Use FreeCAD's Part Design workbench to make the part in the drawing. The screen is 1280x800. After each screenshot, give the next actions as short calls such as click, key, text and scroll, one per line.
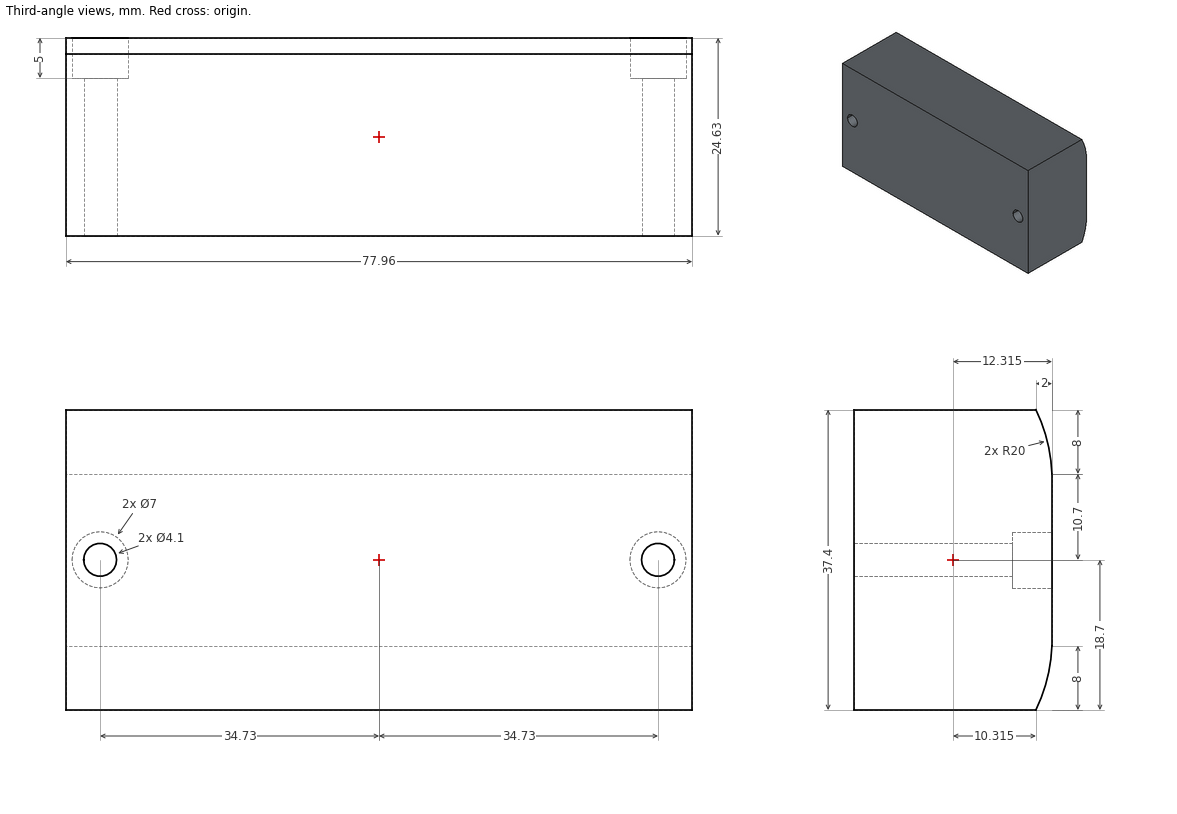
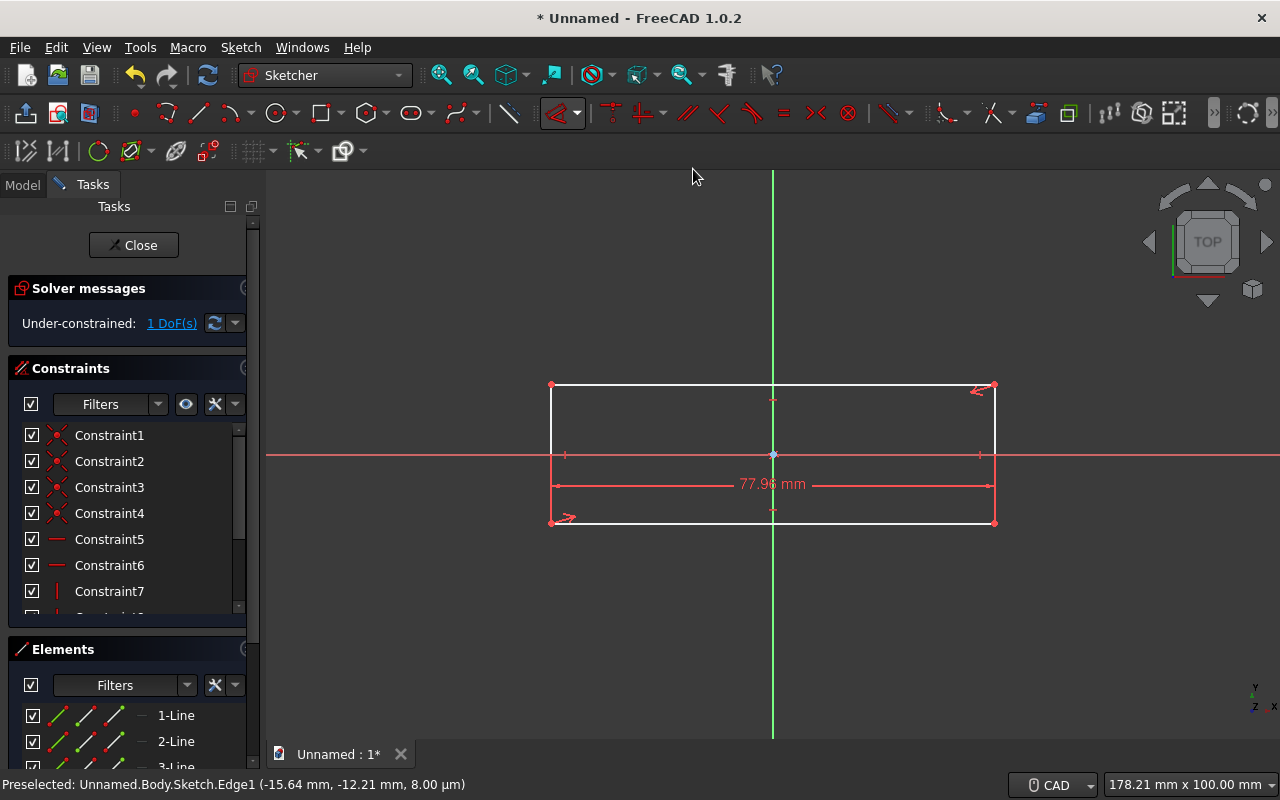
click(995, 482)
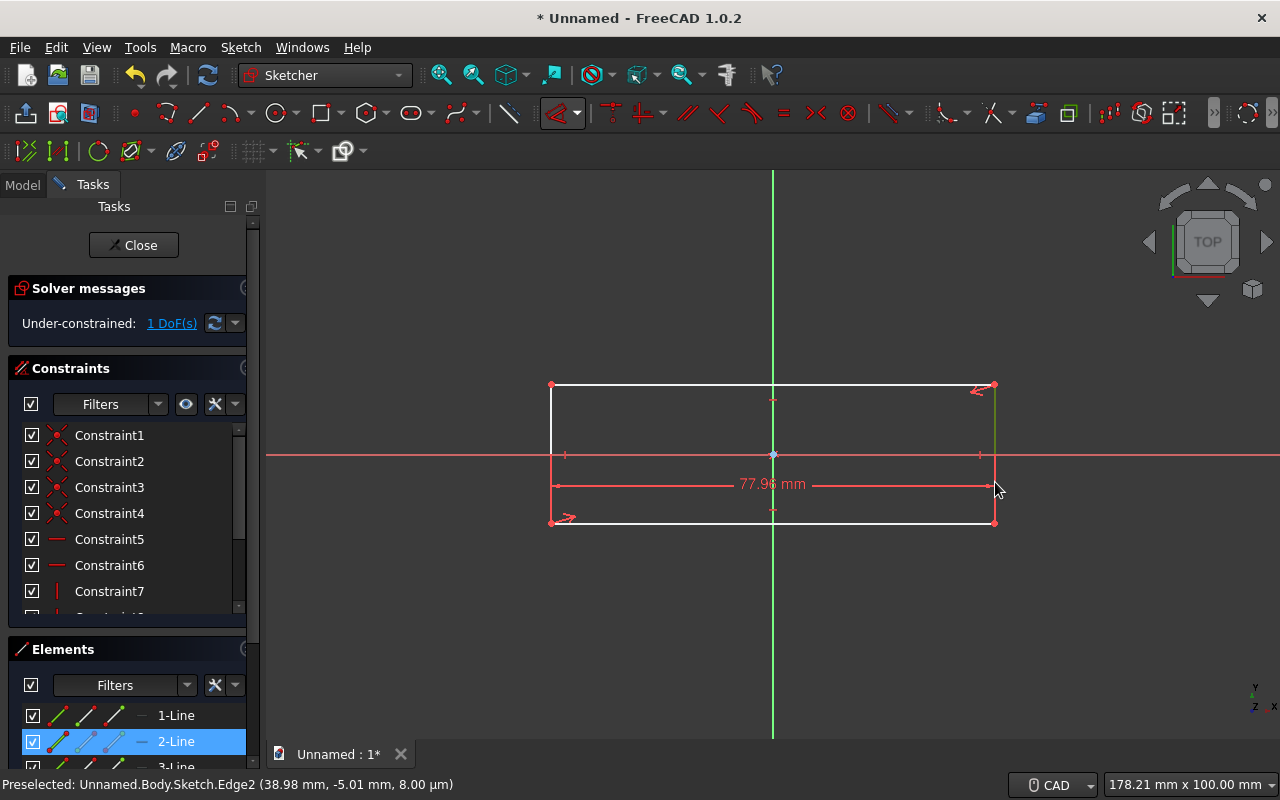
click(580, 114)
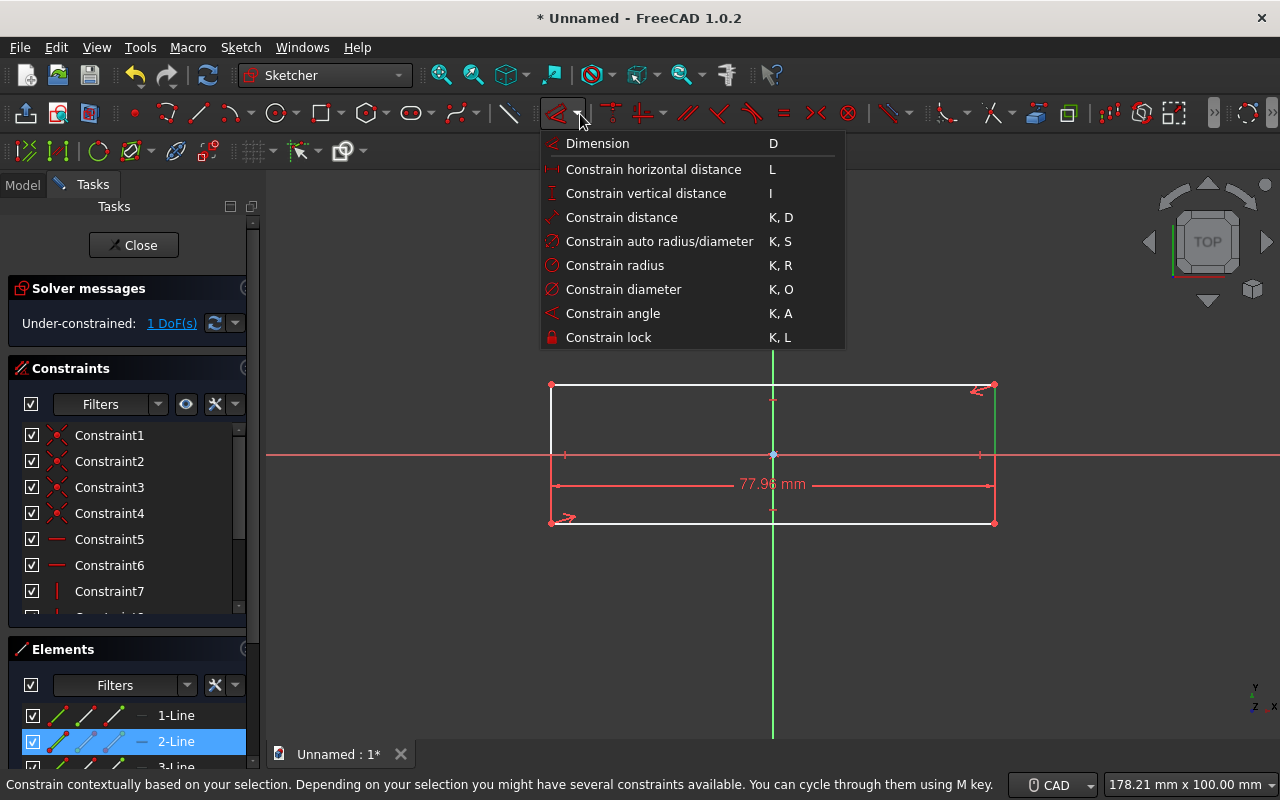
click(693, 193)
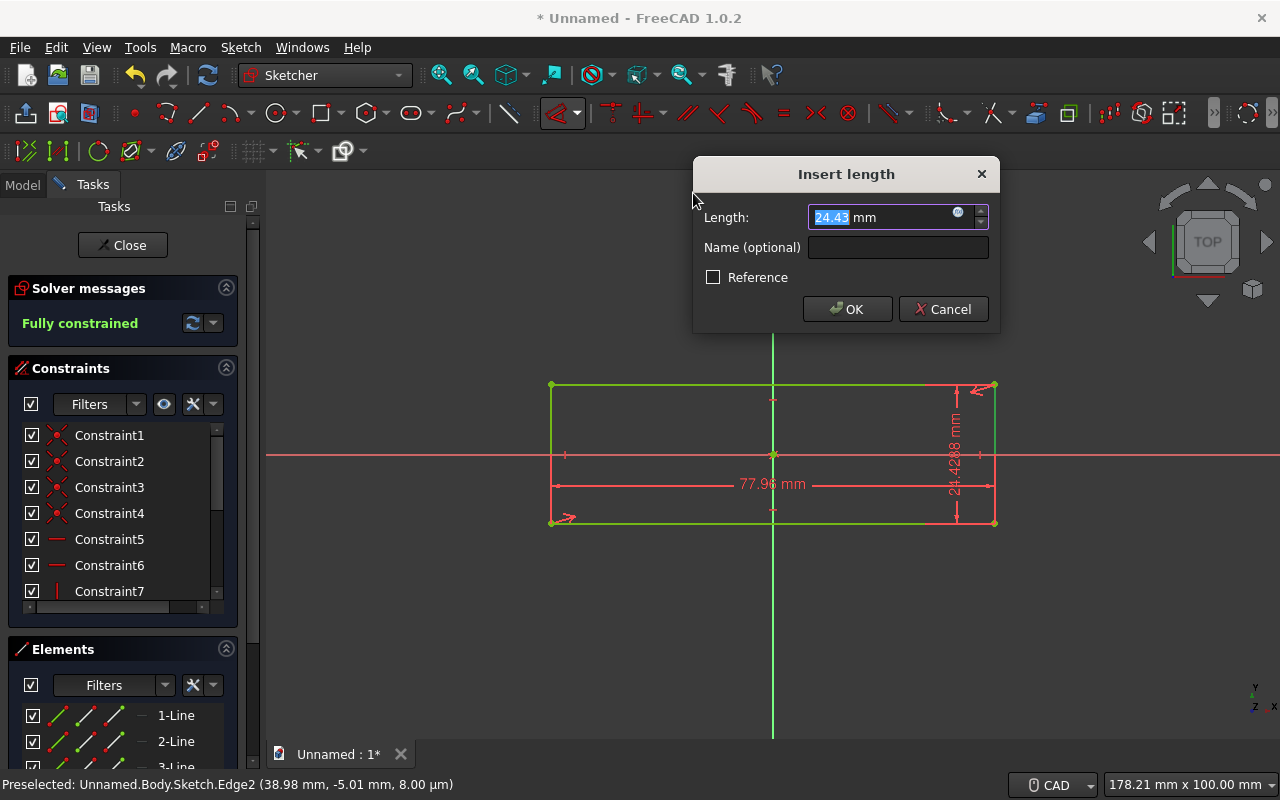
text(24.63)
key(Return)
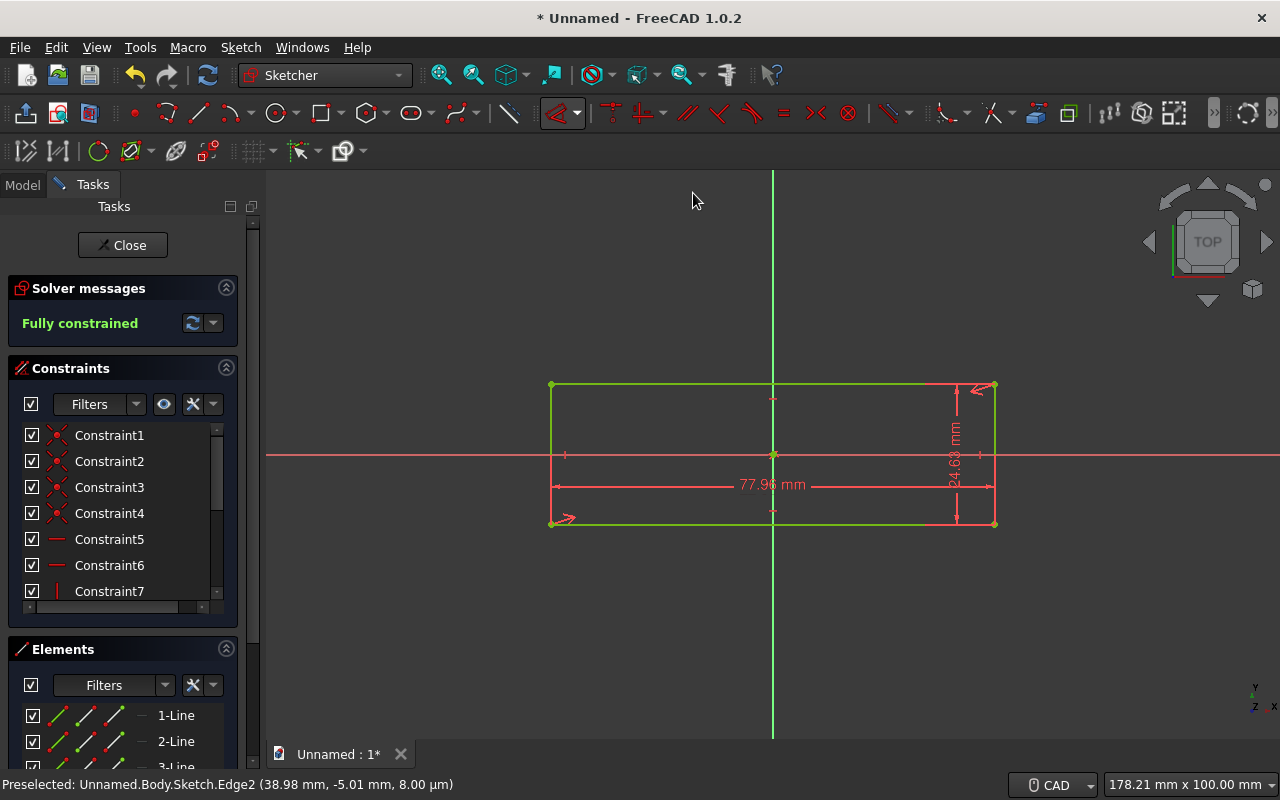
click(123, 245)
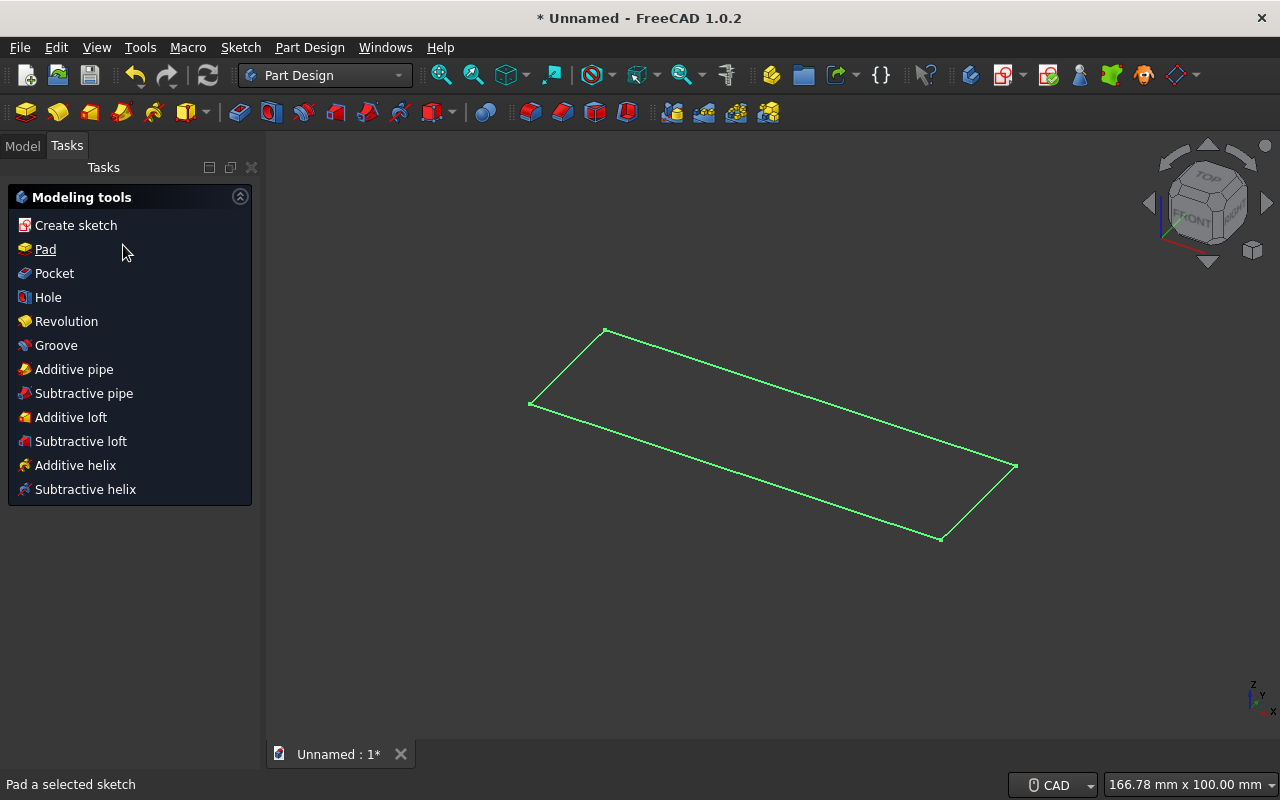
click(26, 112)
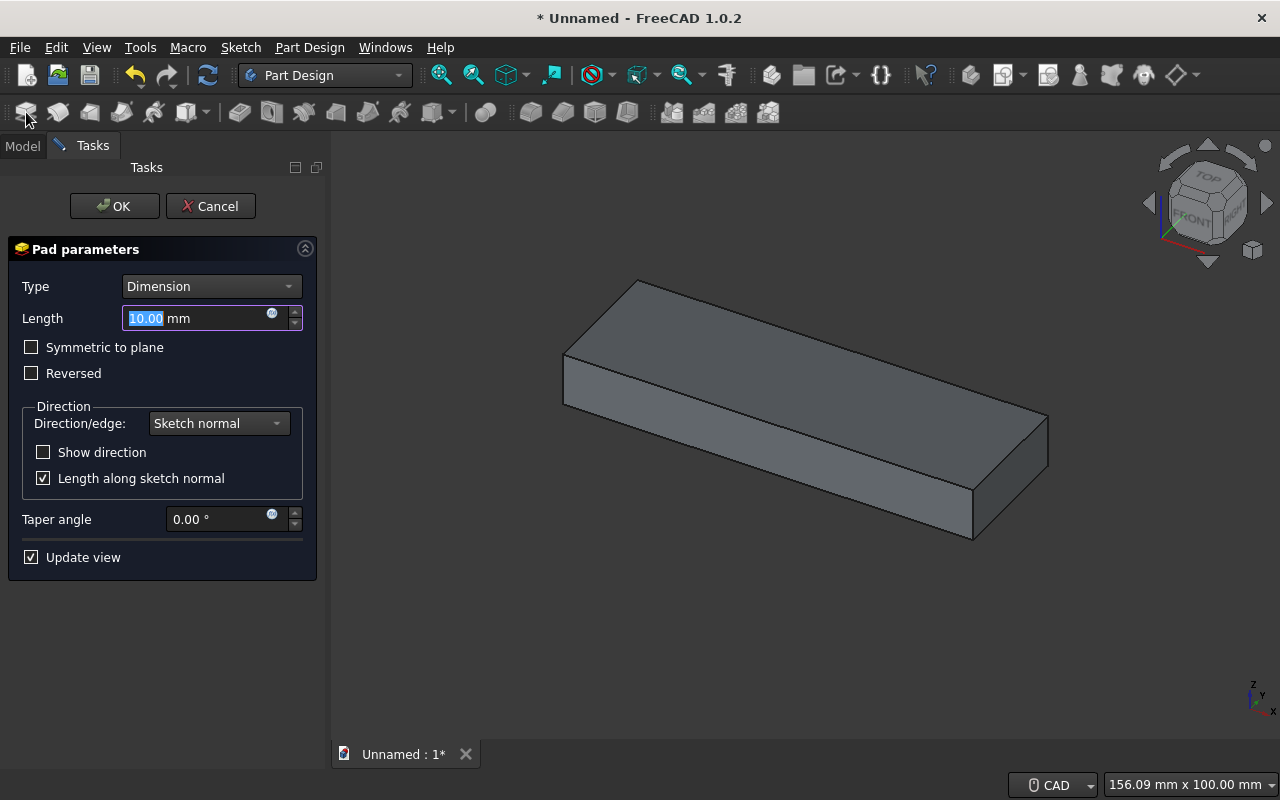
text(37.4)
key(Tab)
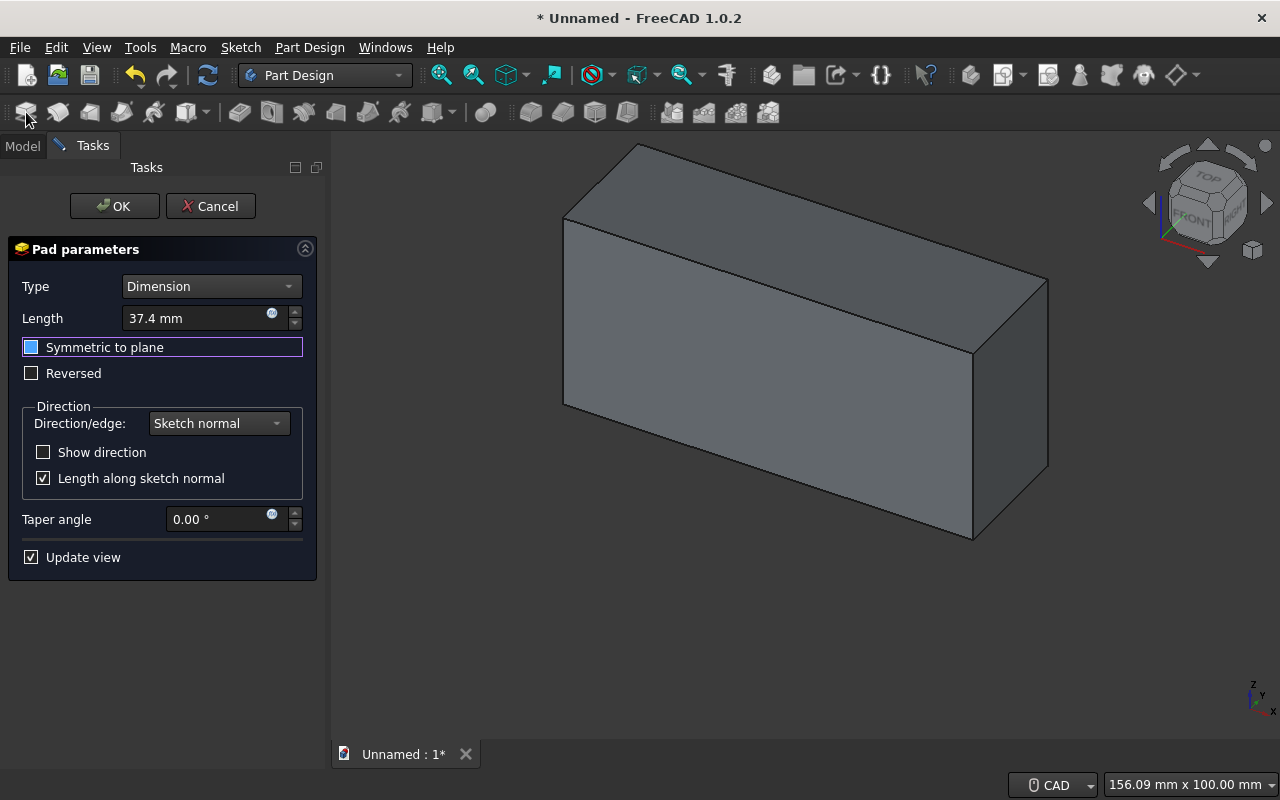
click(30, 347)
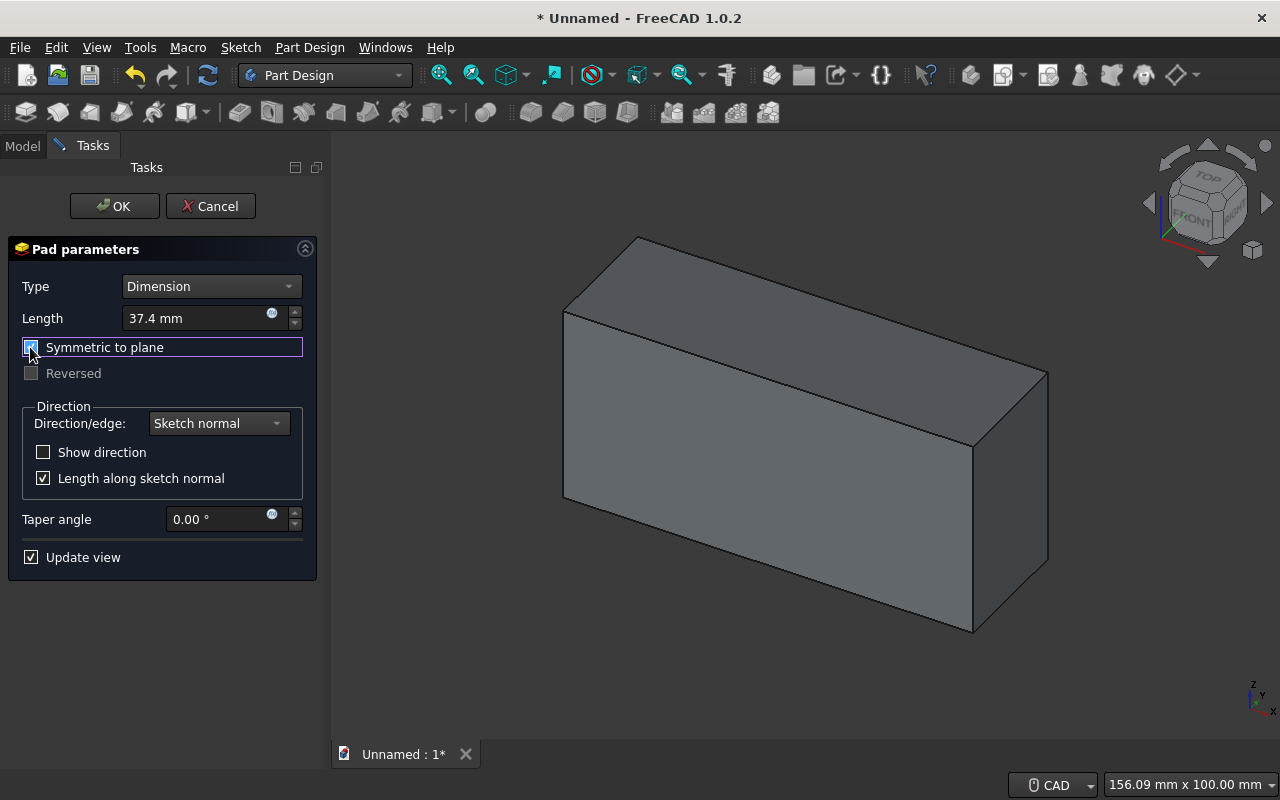
click(115, 206)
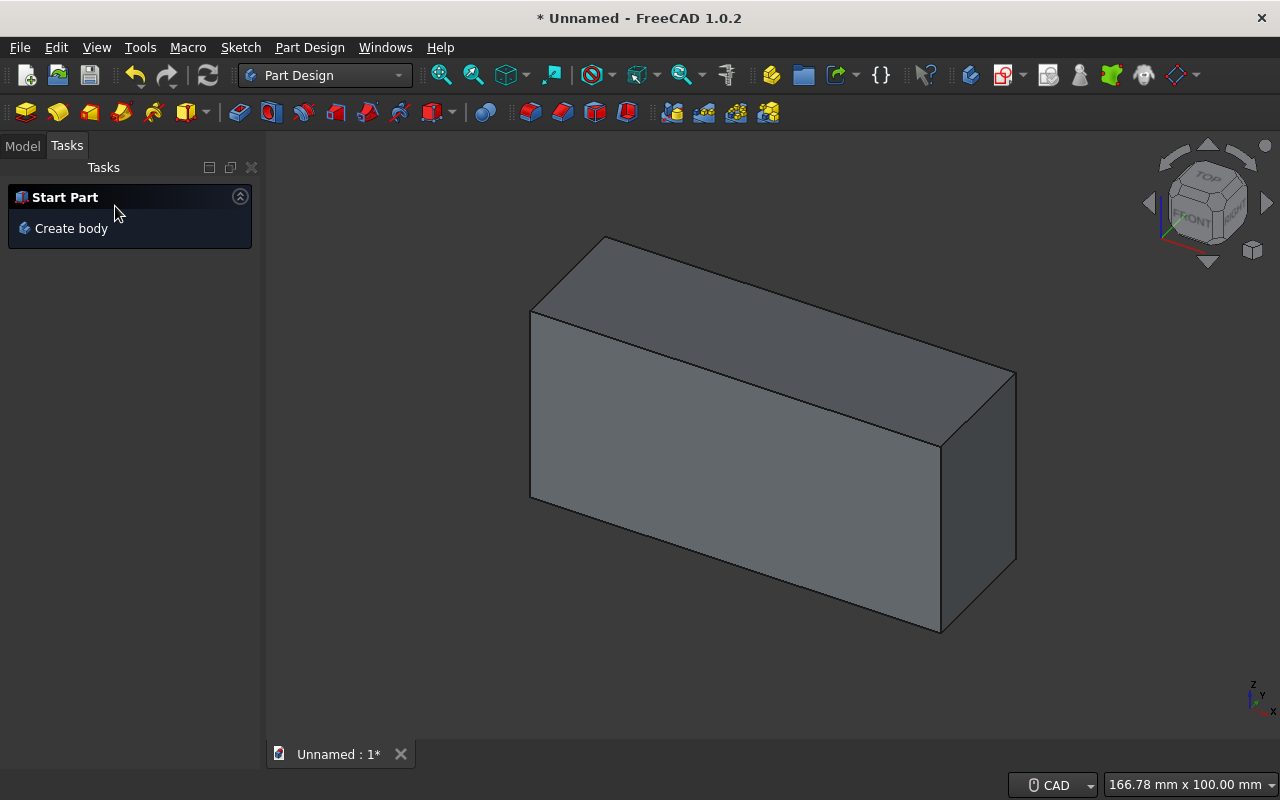
click(978, 475)